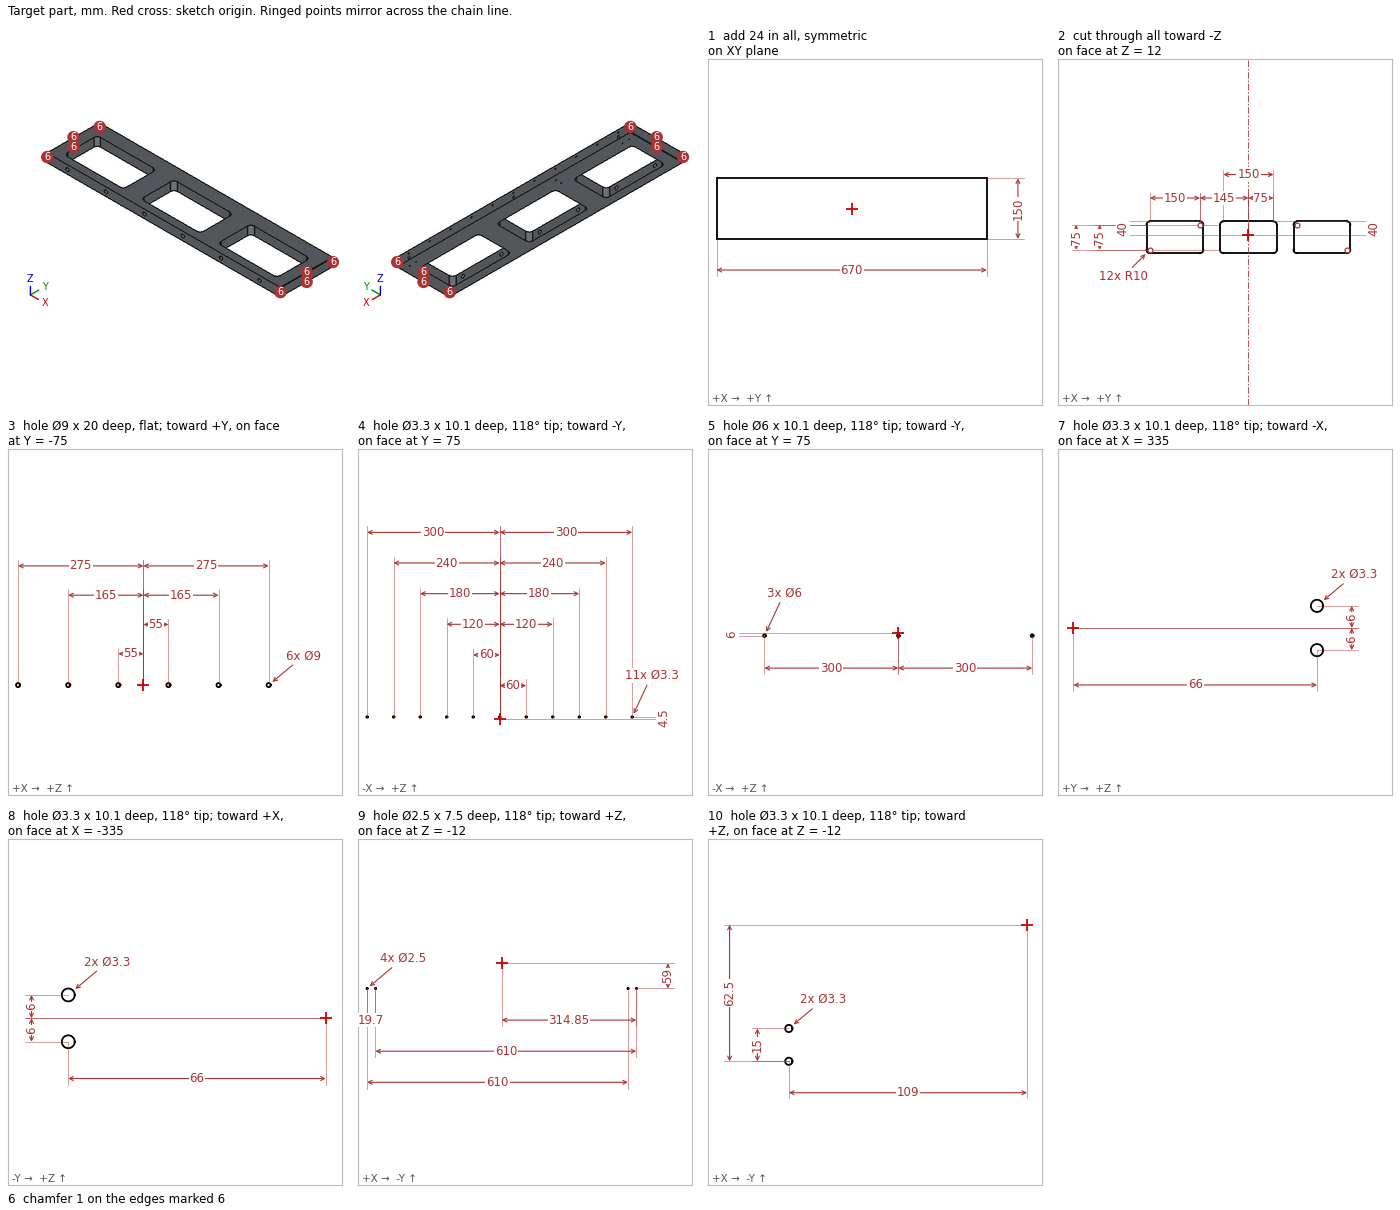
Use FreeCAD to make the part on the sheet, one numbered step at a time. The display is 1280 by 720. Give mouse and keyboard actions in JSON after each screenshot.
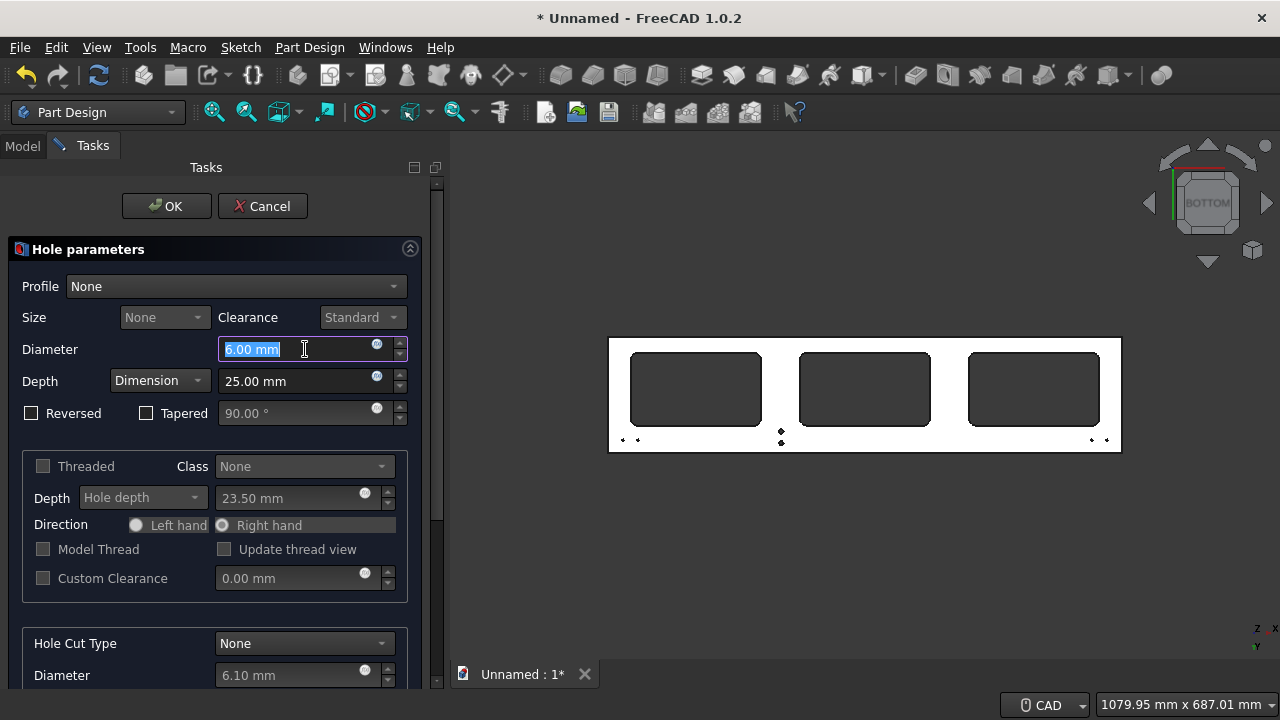
{"action": "type", "text": "3.3"}
{"action": "key", "text": "Tab"}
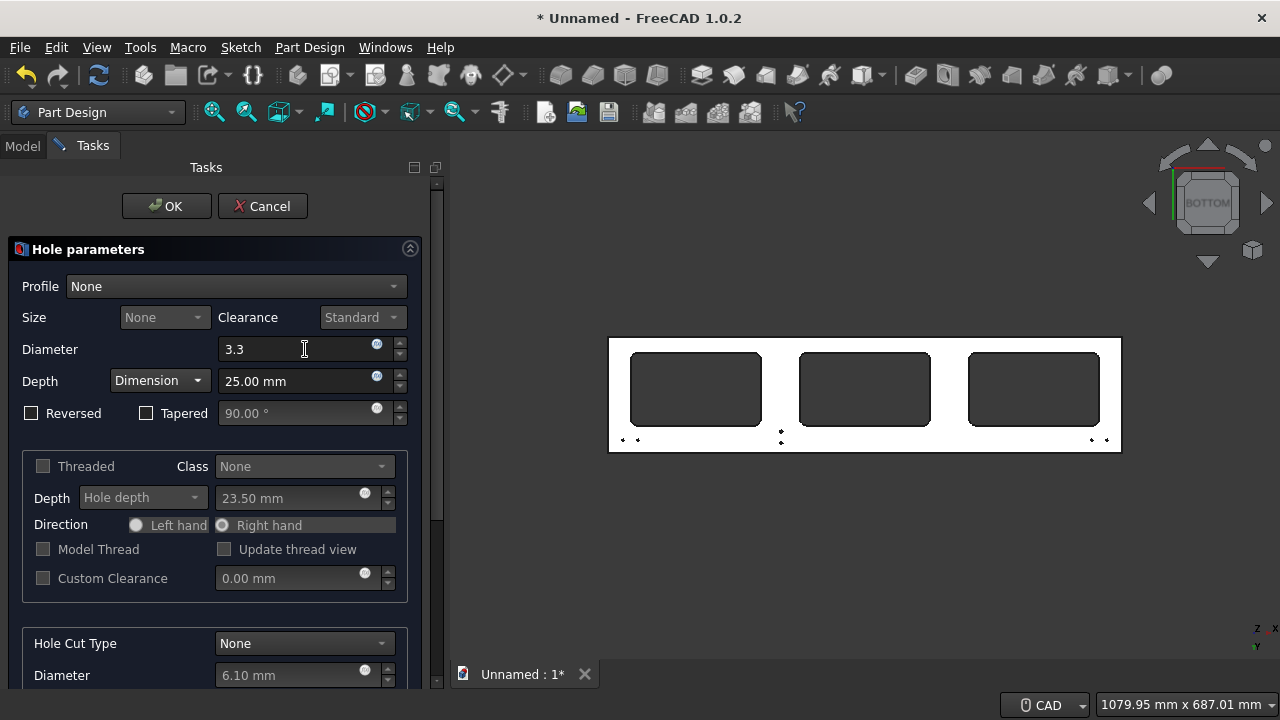
{"action": "triple_click", "coordinate": [305, 381]}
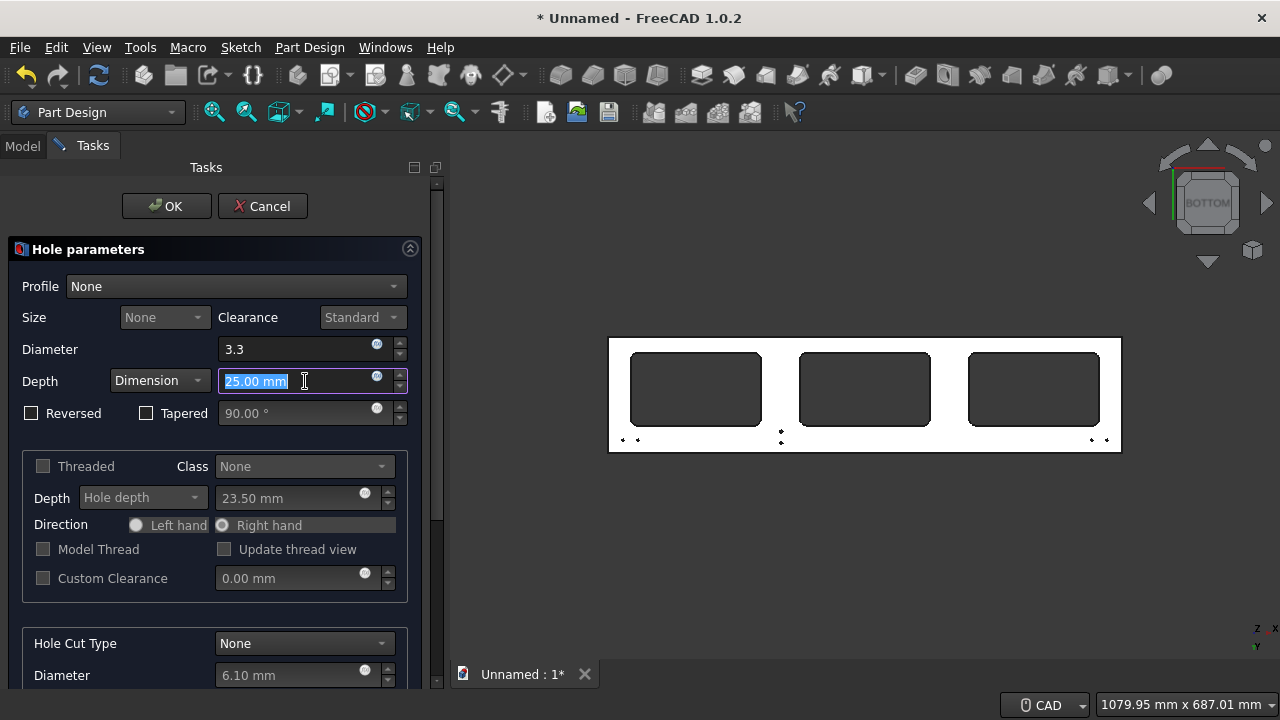
{"action": "type", "text": "10.1"}
{"action": "key", "text": "Tab"}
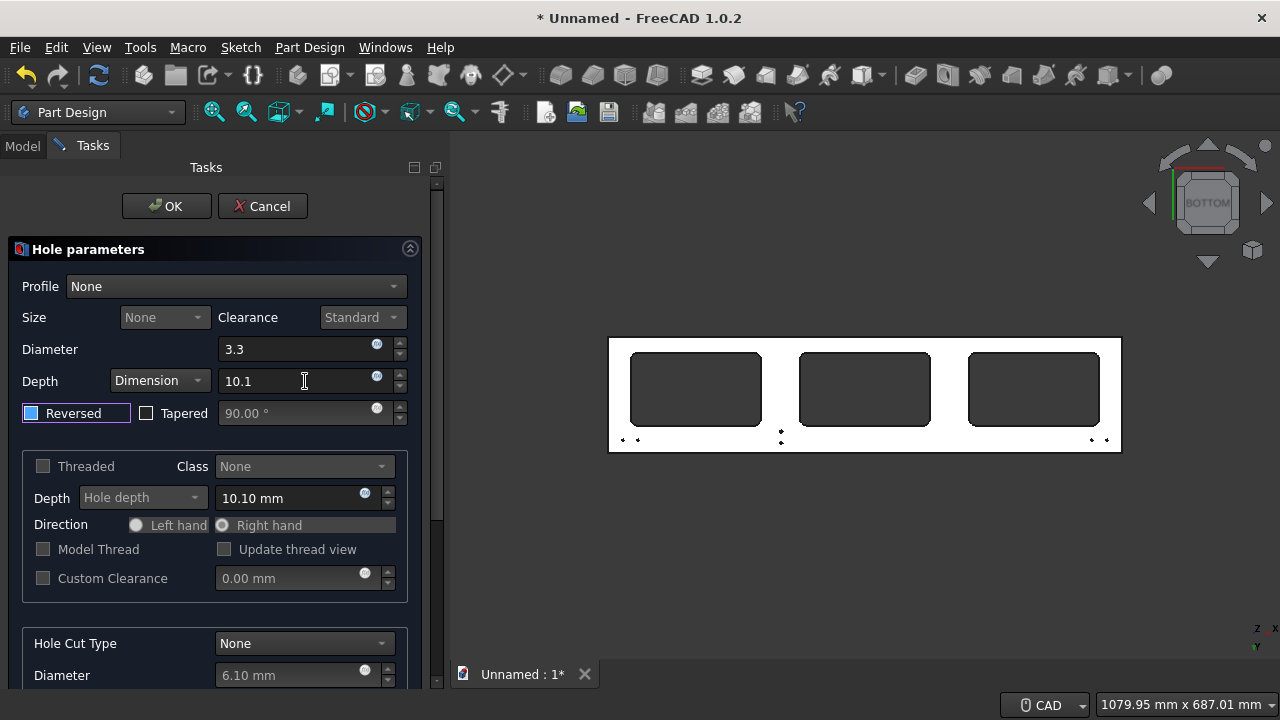
{"action": "left_click", "coordinate": [167, 206]}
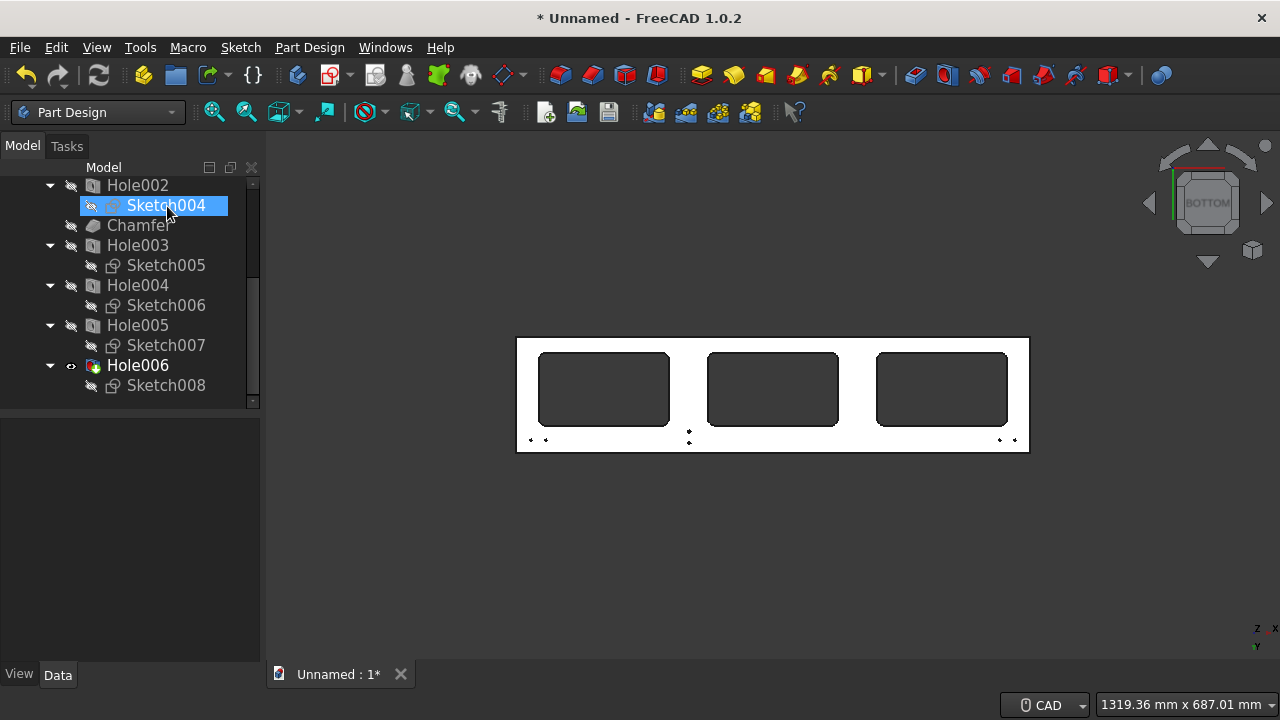
{"action": "key", "text": "0"}